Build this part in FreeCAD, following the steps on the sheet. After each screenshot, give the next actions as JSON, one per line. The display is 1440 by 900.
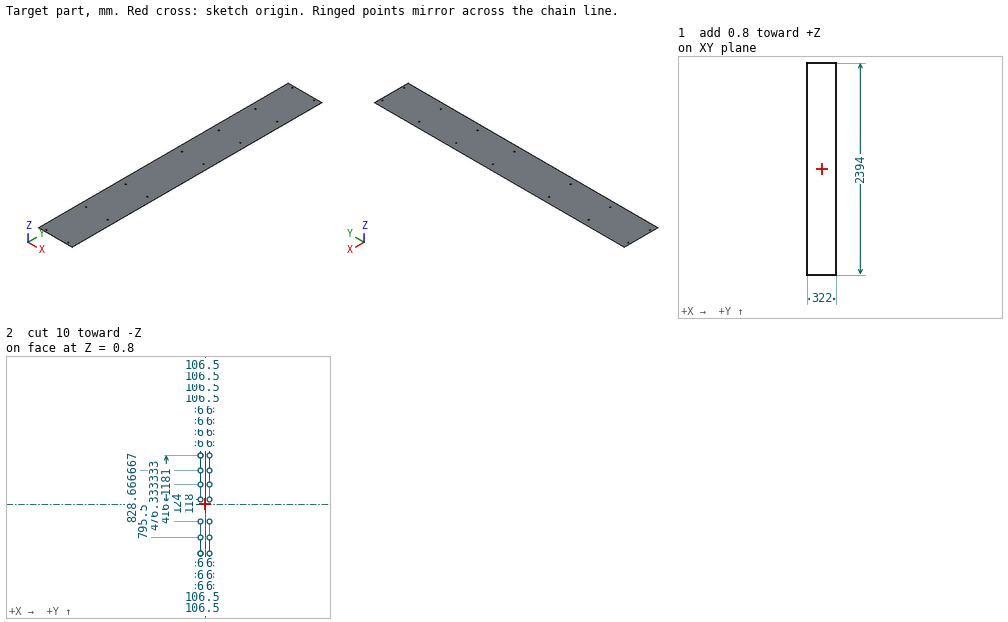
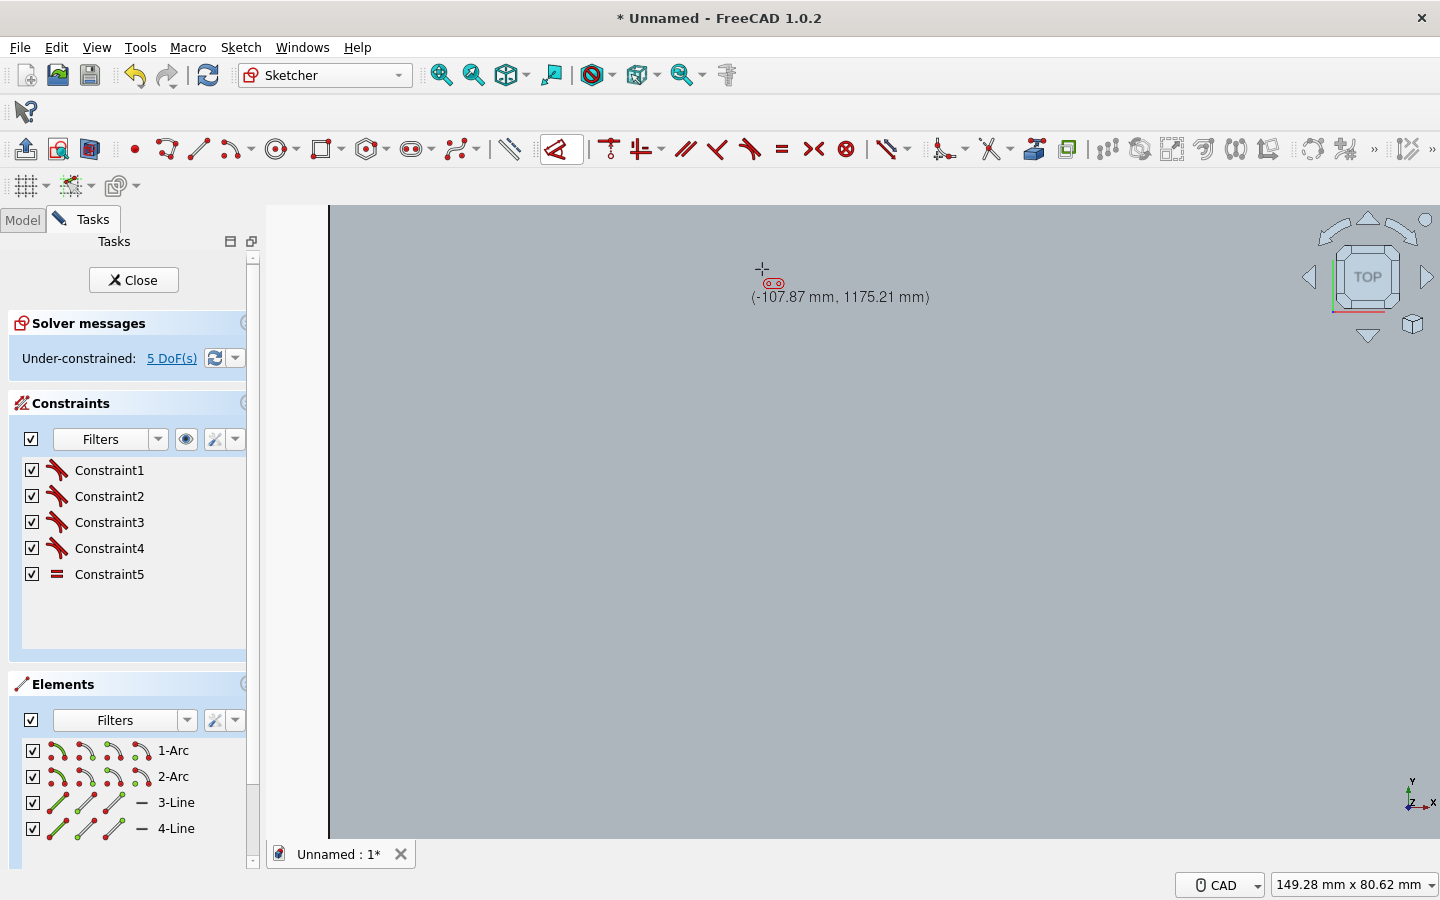
{"action": "scroll", "coordinate": [762, 269], "scroll_direction": "down", "scroll_amount": 18}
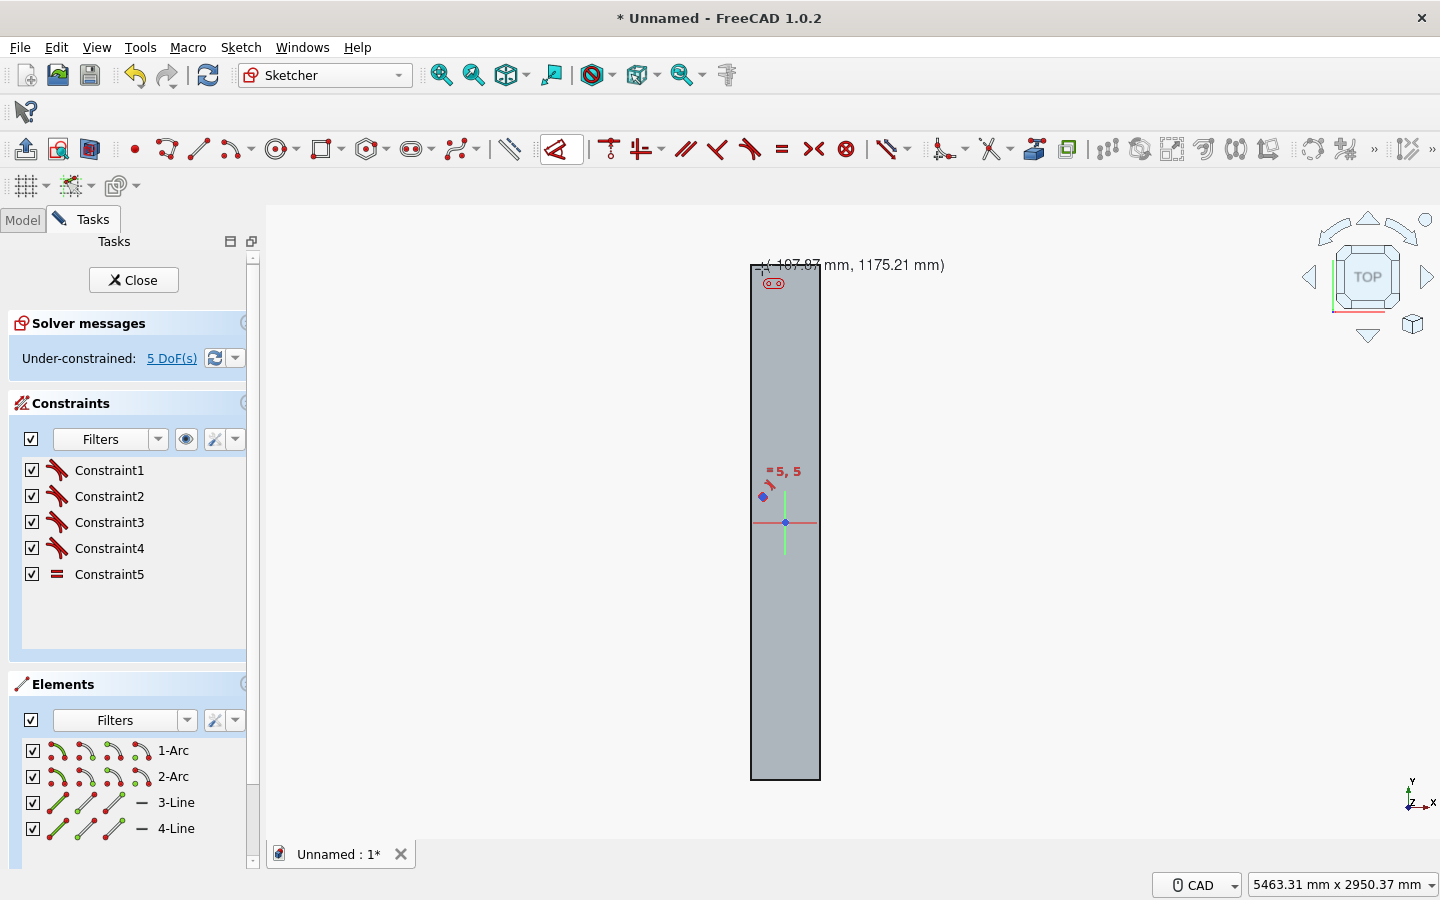
{"action": "left_click", "coordinate": [762, 269]}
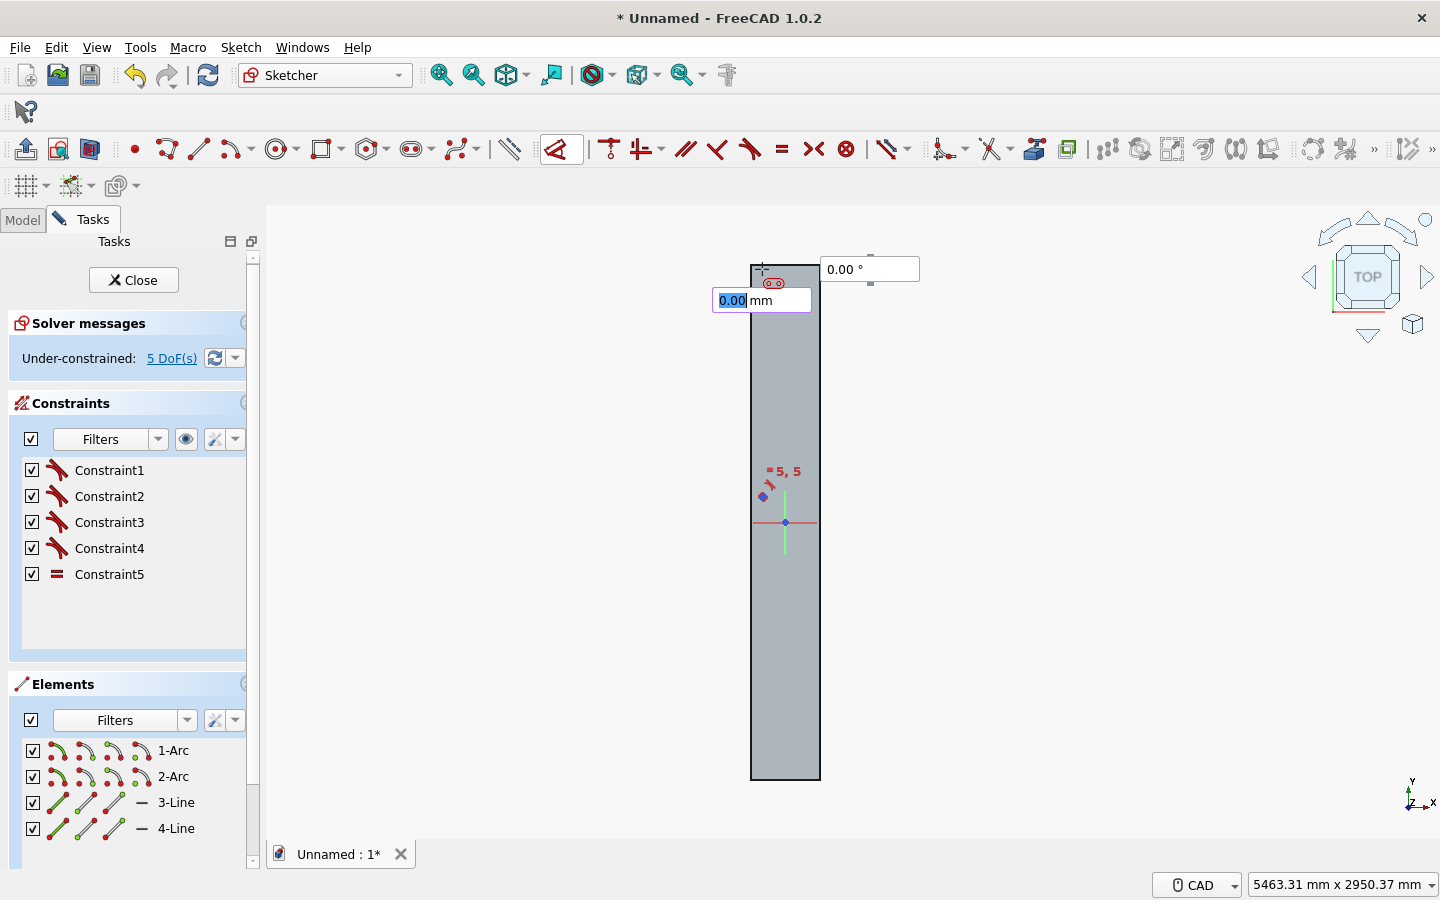
{"action": "scroll", "coordinate": [764, 269], "scroll_direction": "up", "scroll_amount": 13}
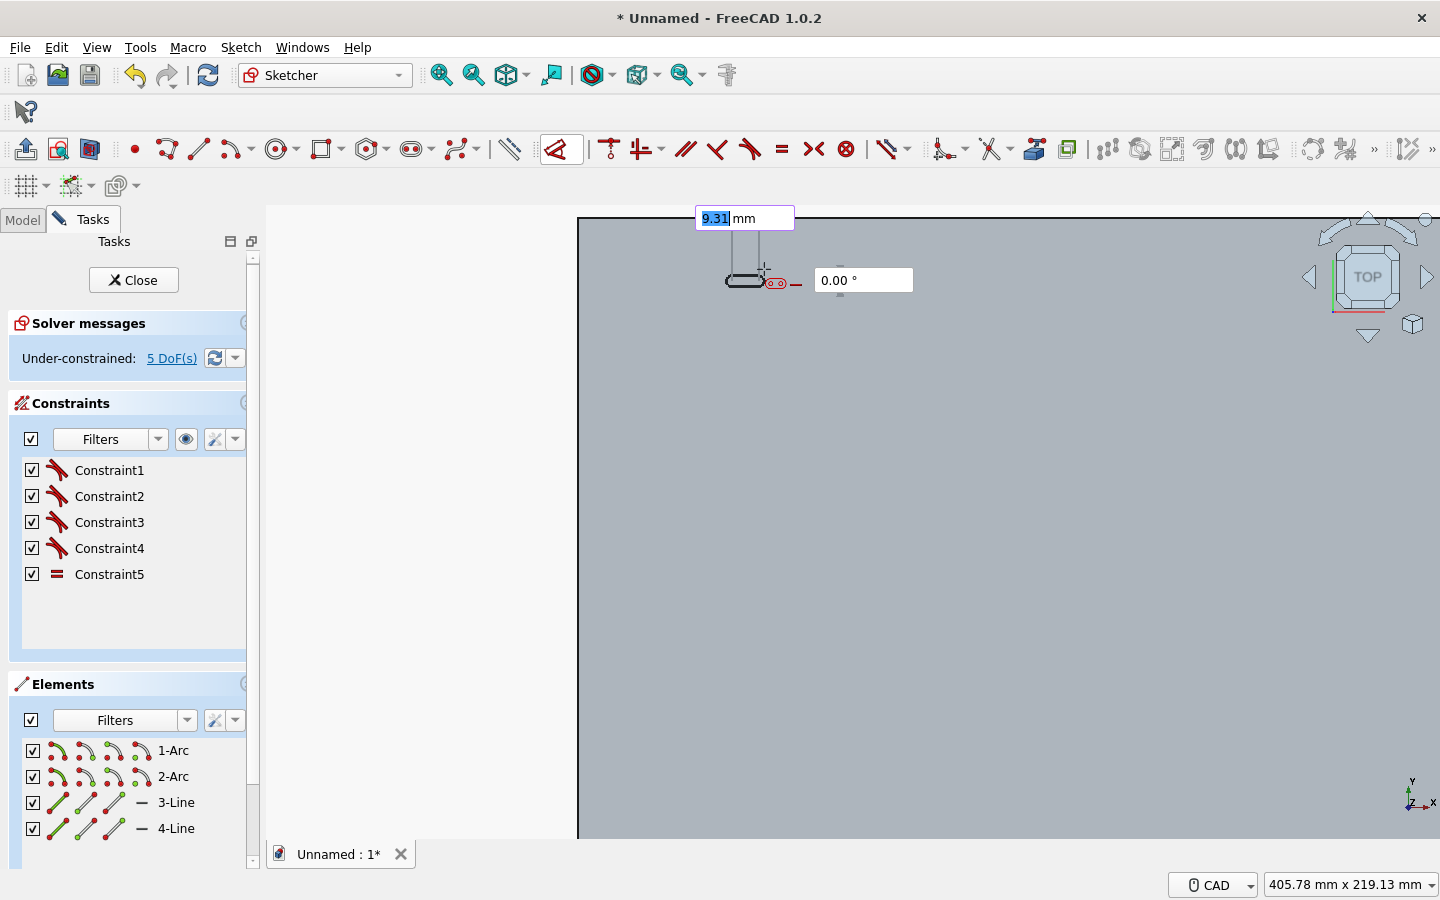
{"action": "left_click", "coordinate": [753, 268]}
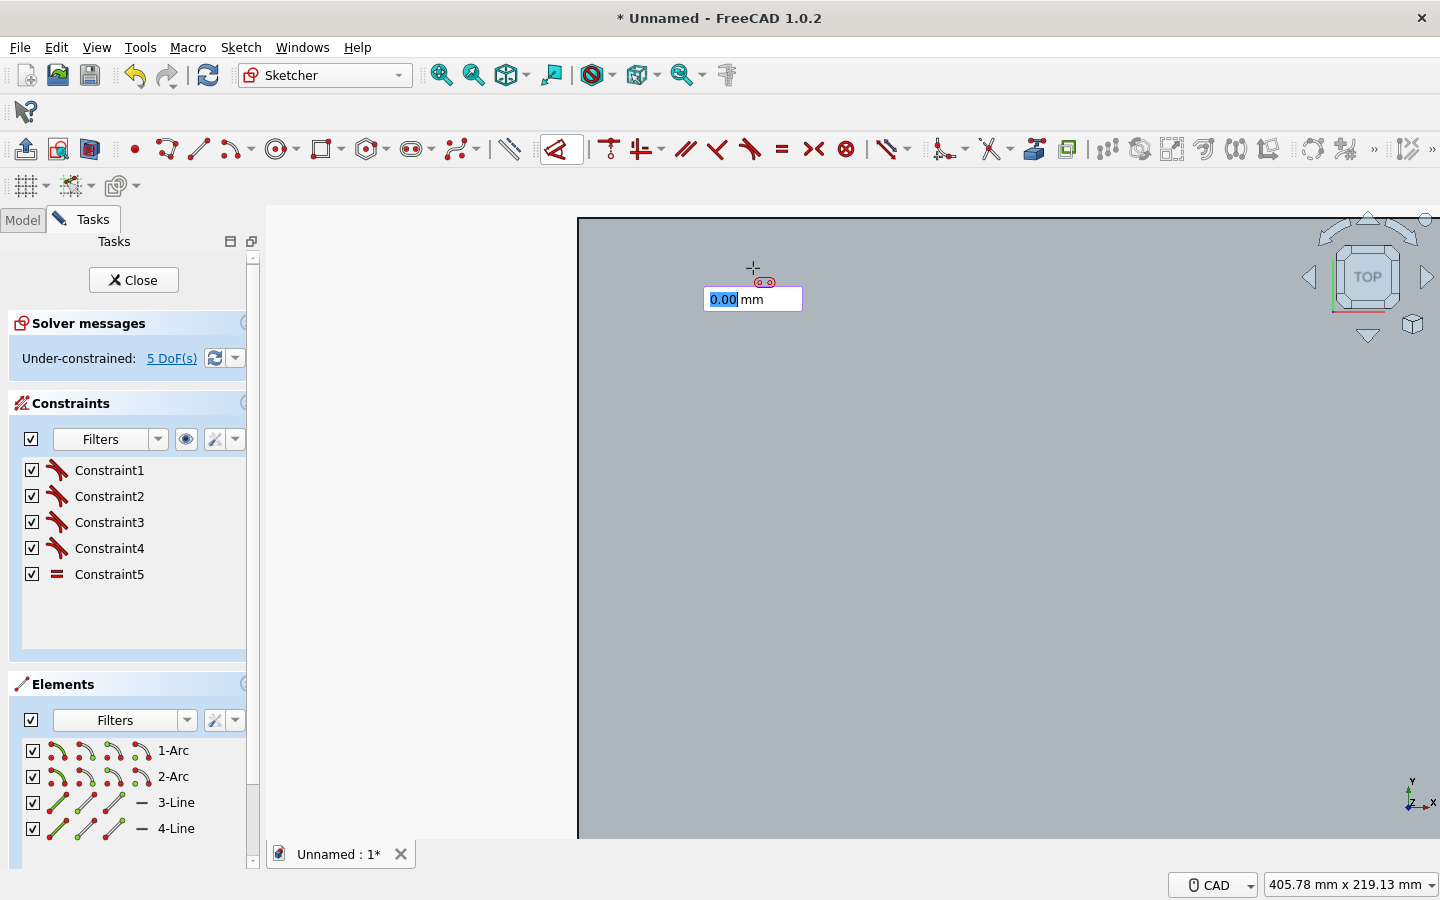
{"action": "scroll", "coordinate": [744, 264], "scroll_direction": "up", "scroll_amount": 4}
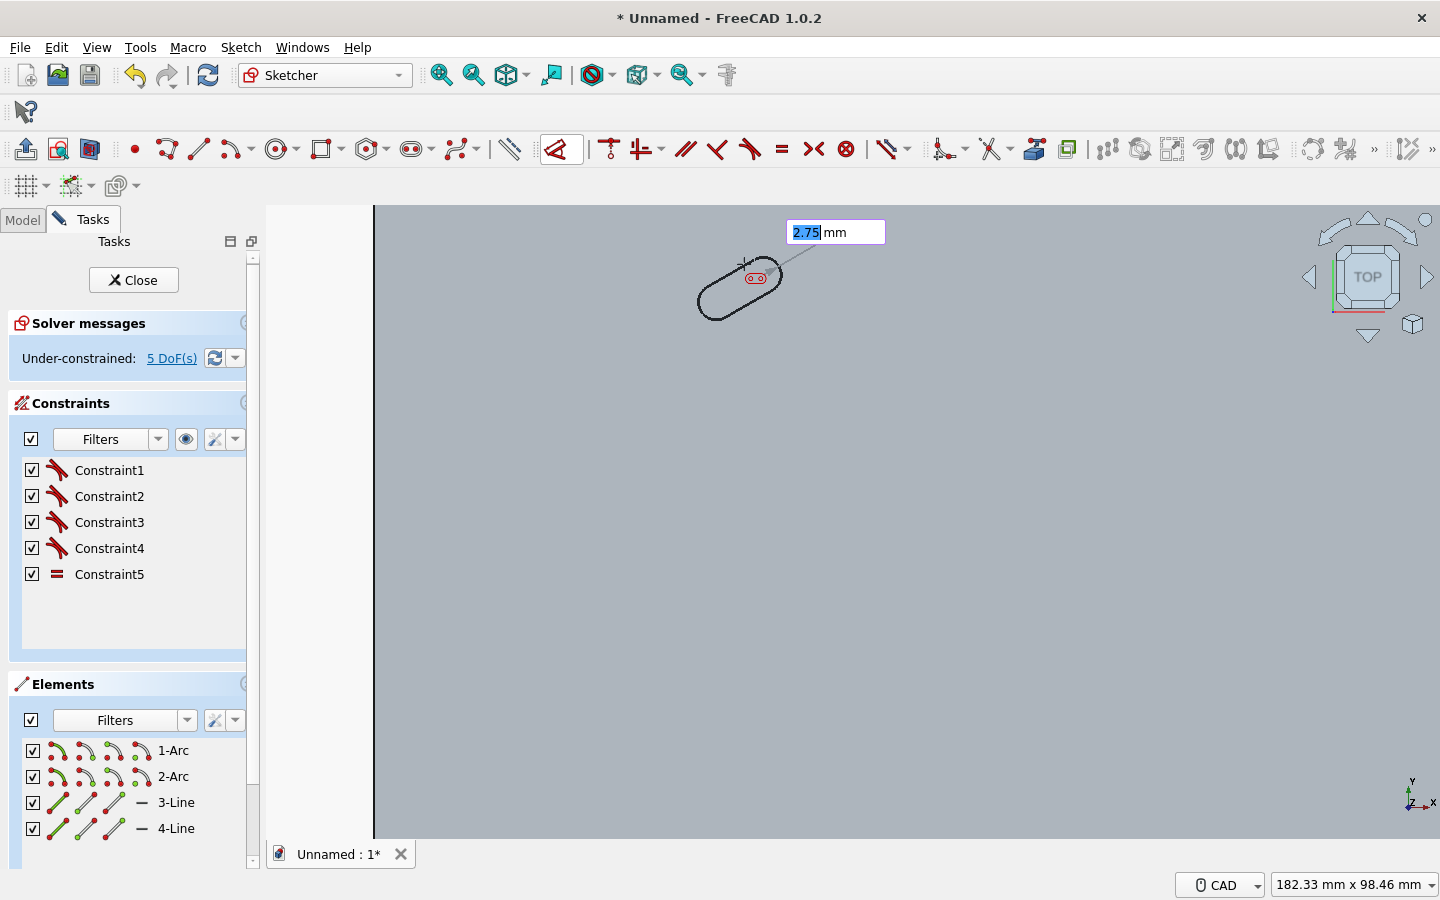
{"action": "left_click", "coordinate": [744, 265]}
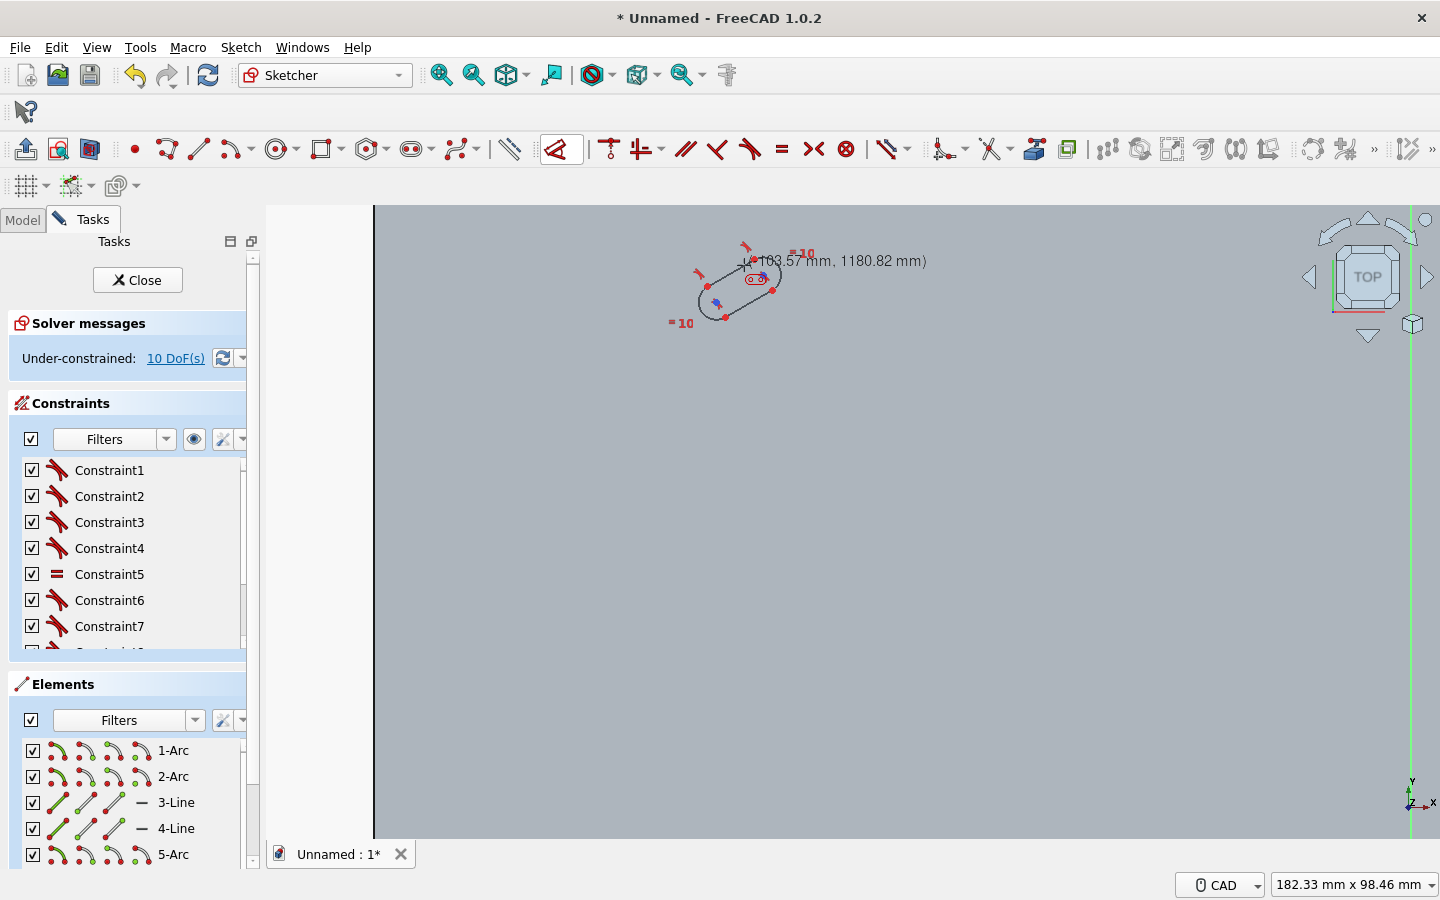
{"action": "scroll", "coordinate": [763, 268], "scroll_direction": "down", "scroll_amount": 17}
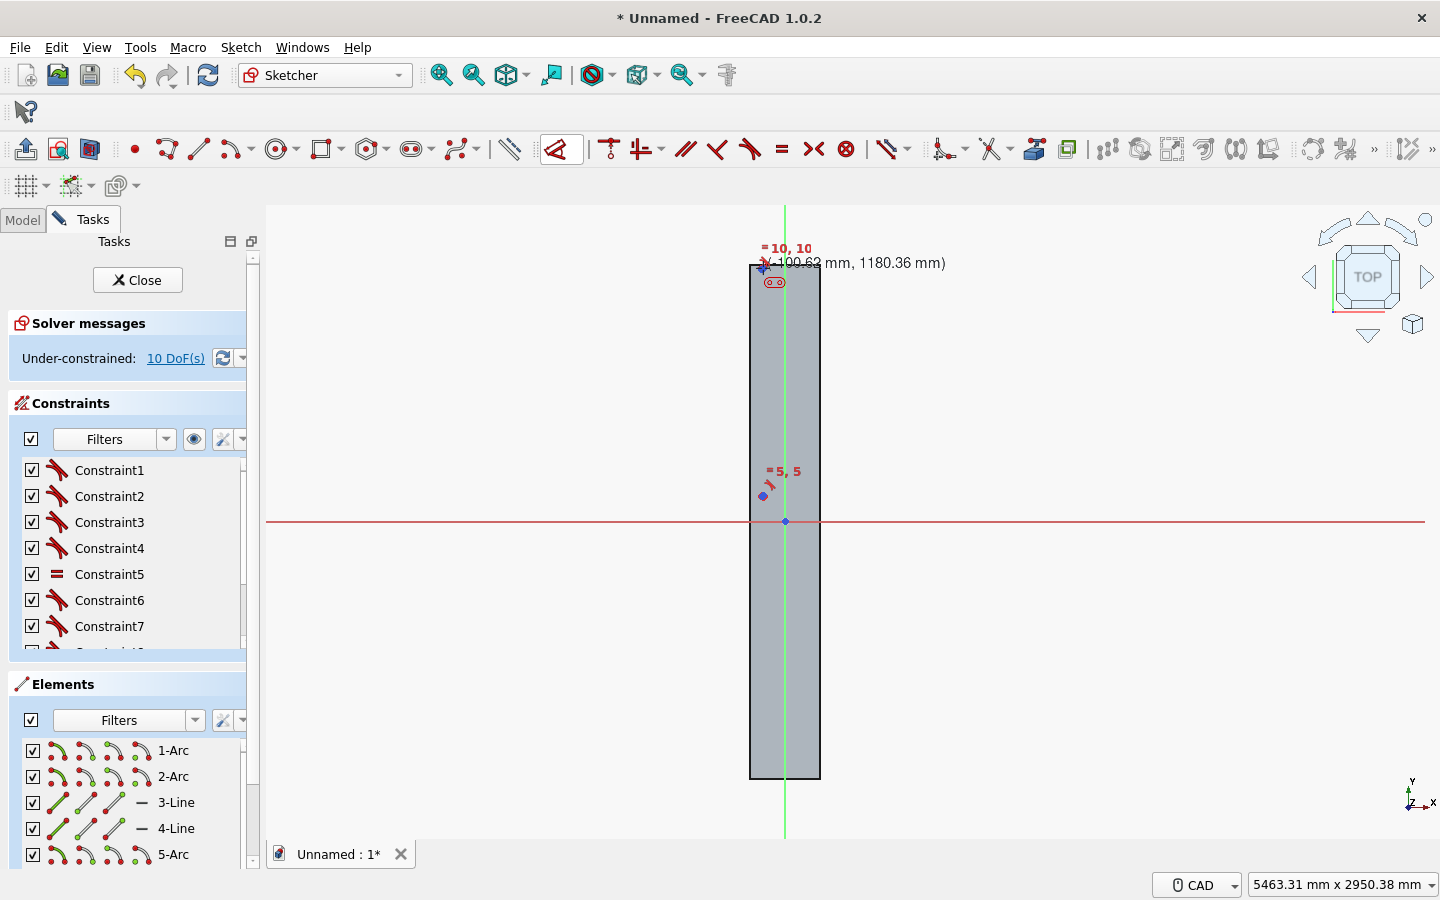
{"action": "scroll", "coordinate": [762, 344], "scroll_direction": "up", "scroll_amount": 18}